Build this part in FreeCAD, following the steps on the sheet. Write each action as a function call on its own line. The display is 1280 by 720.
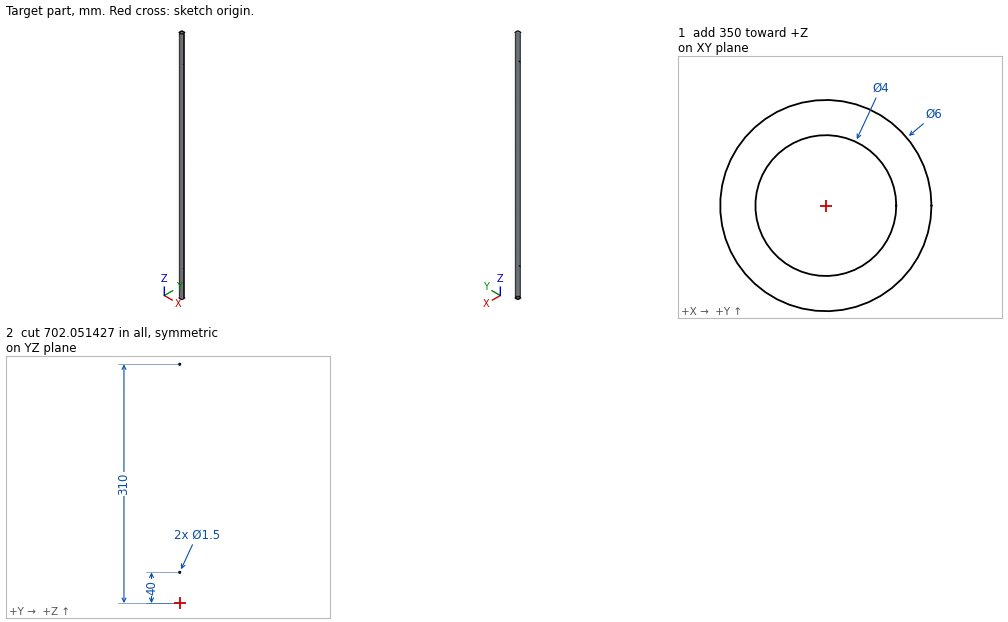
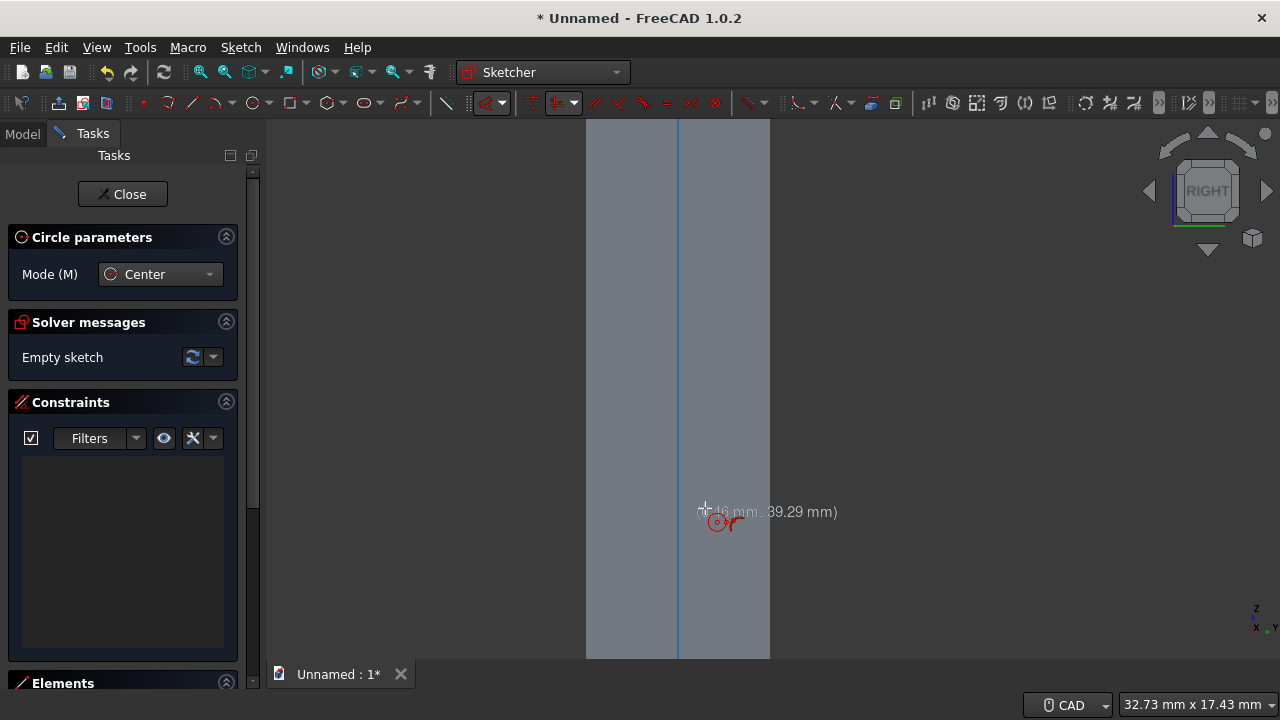
scroll(706, 536, down, 16)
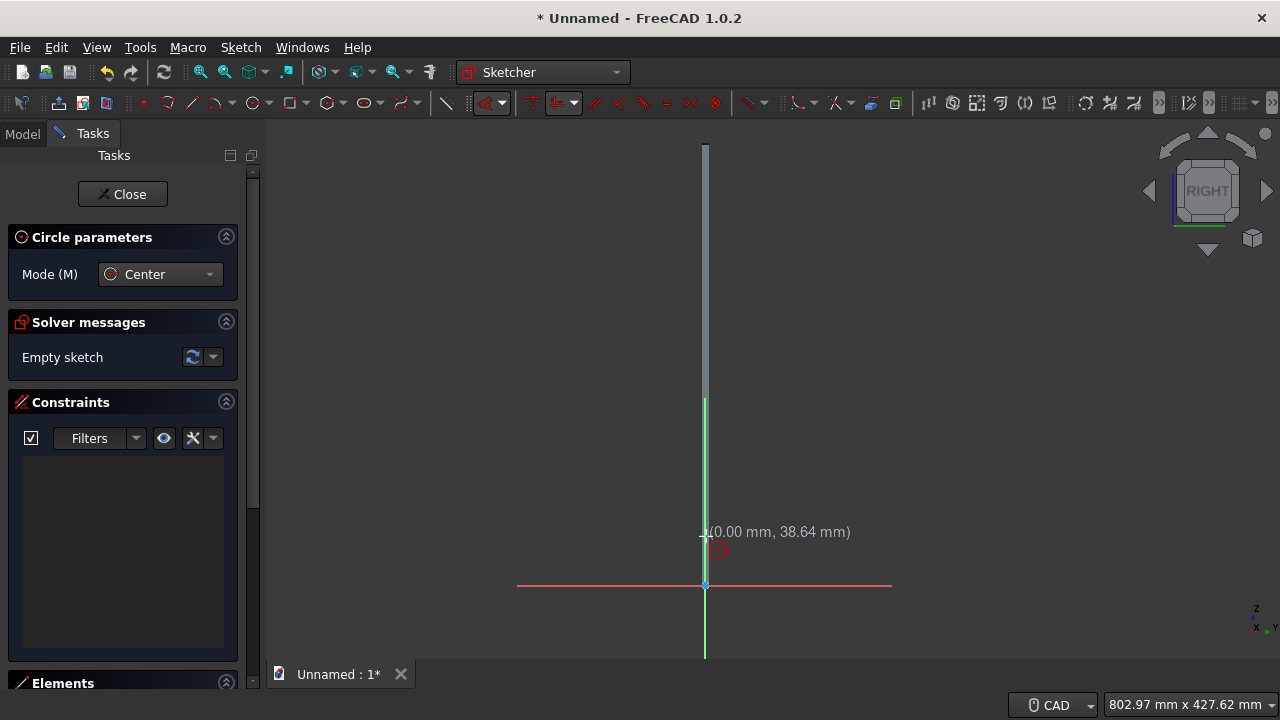
click(705, 535)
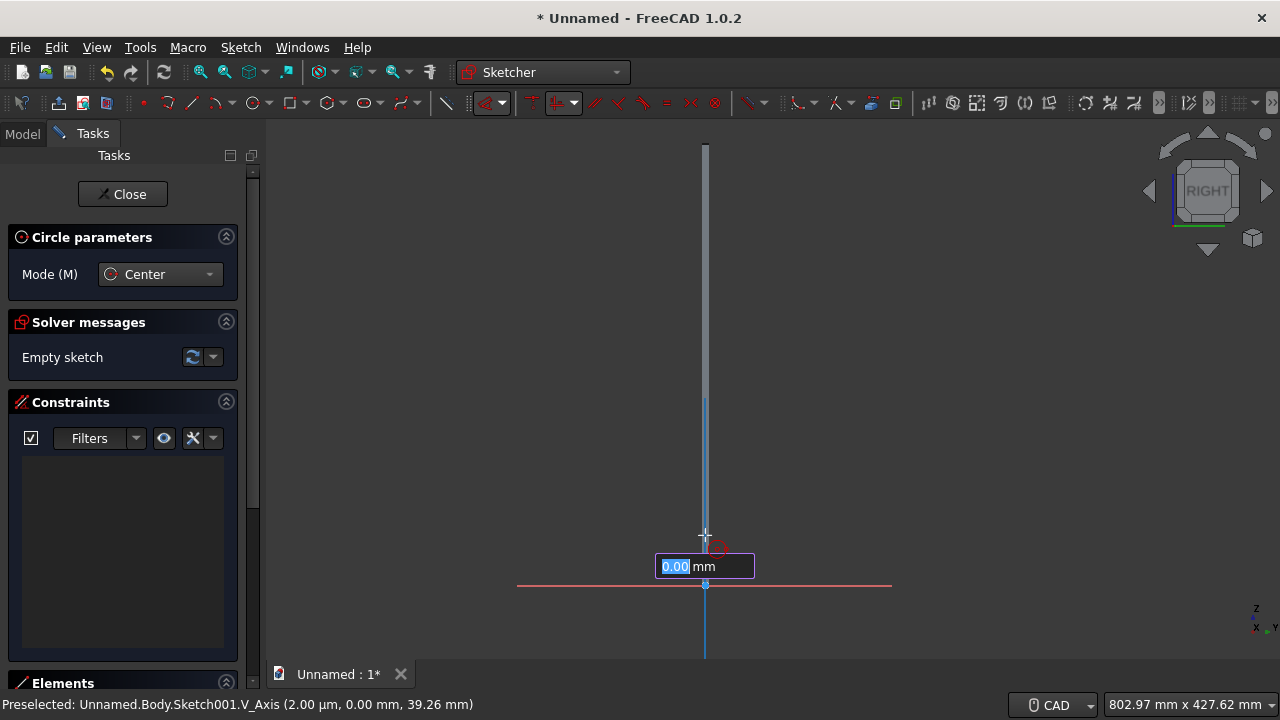
scroll(706, 535, up, 15)
move(701, 515)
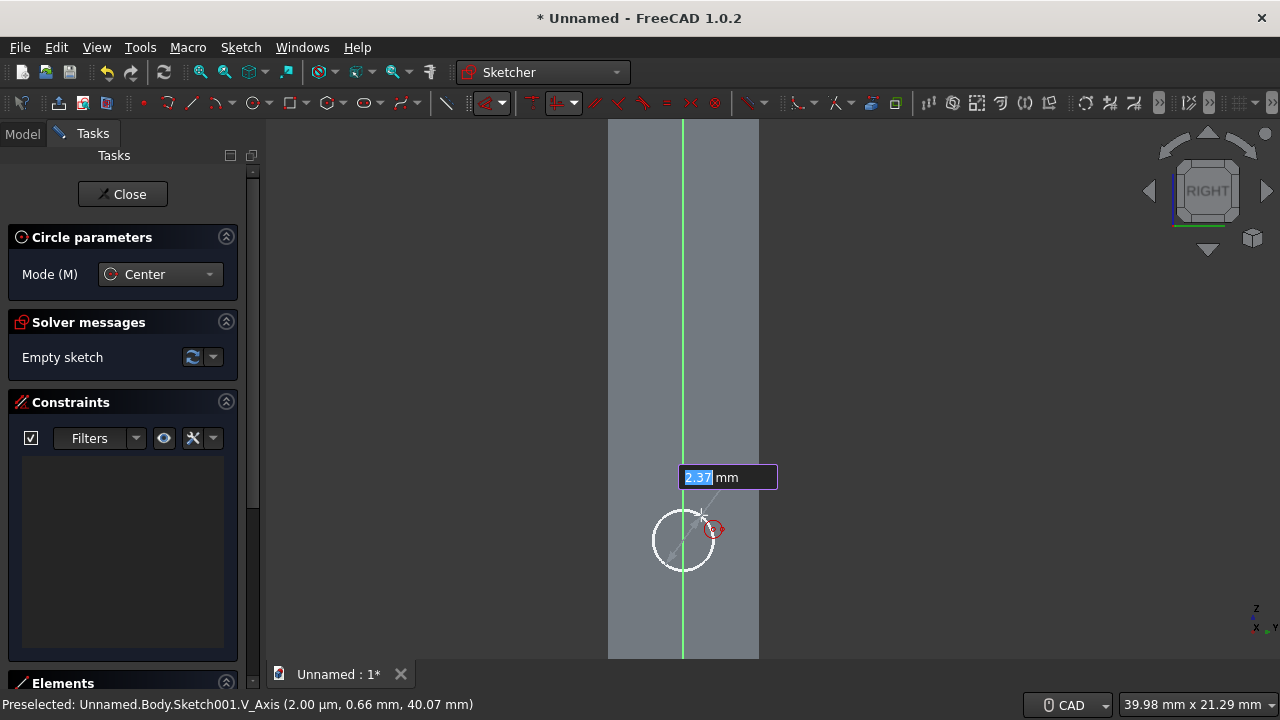
text(1.5)
key(Return)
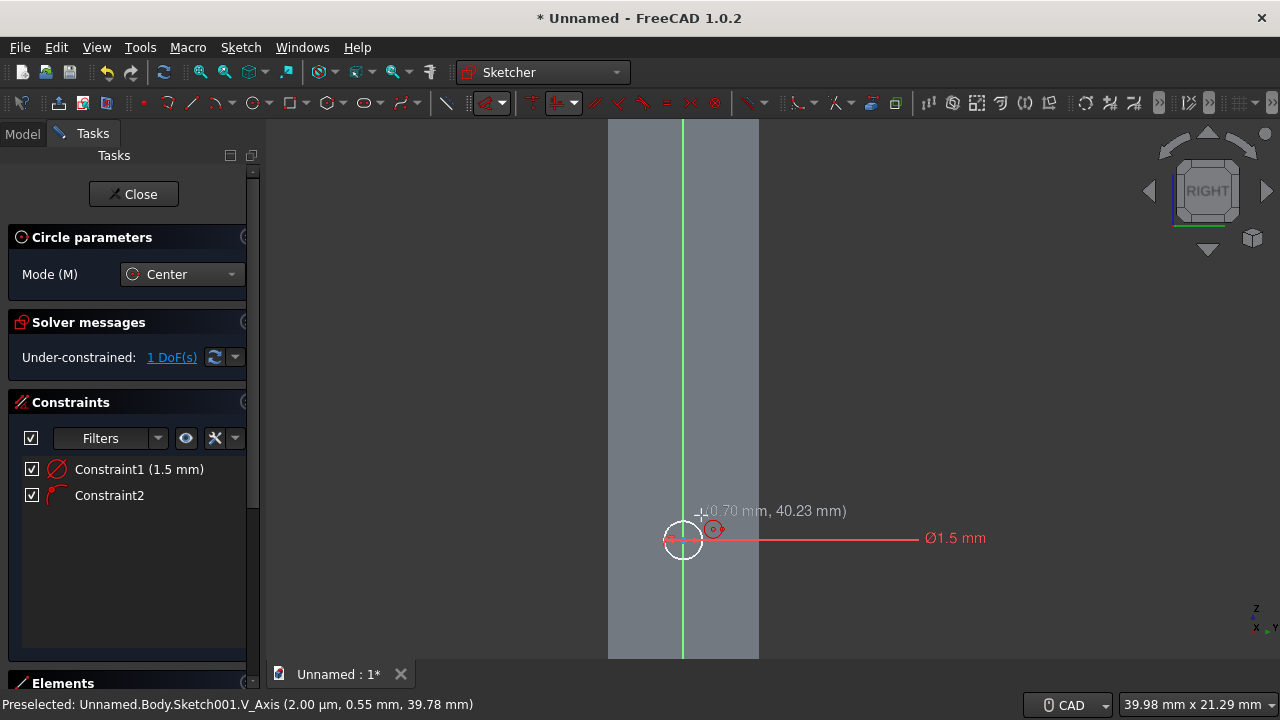
scroll(706, 535, down, 15)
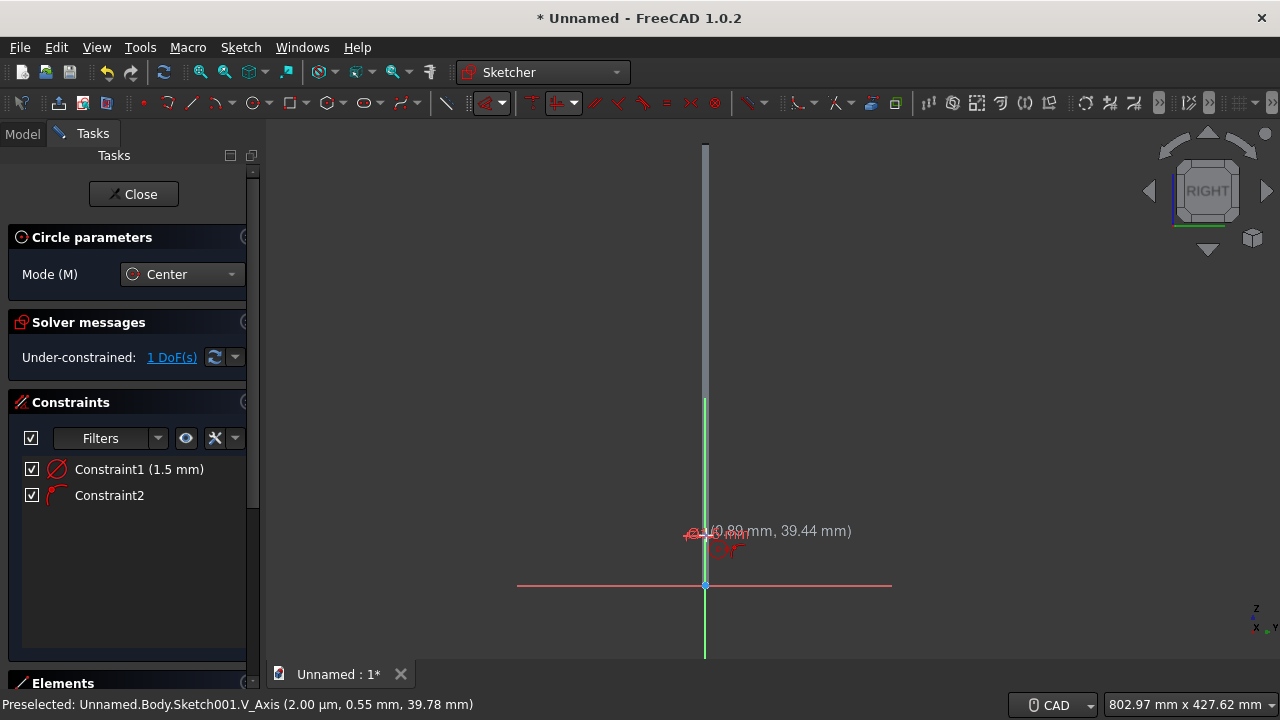
scroll(705, 194, up, 16)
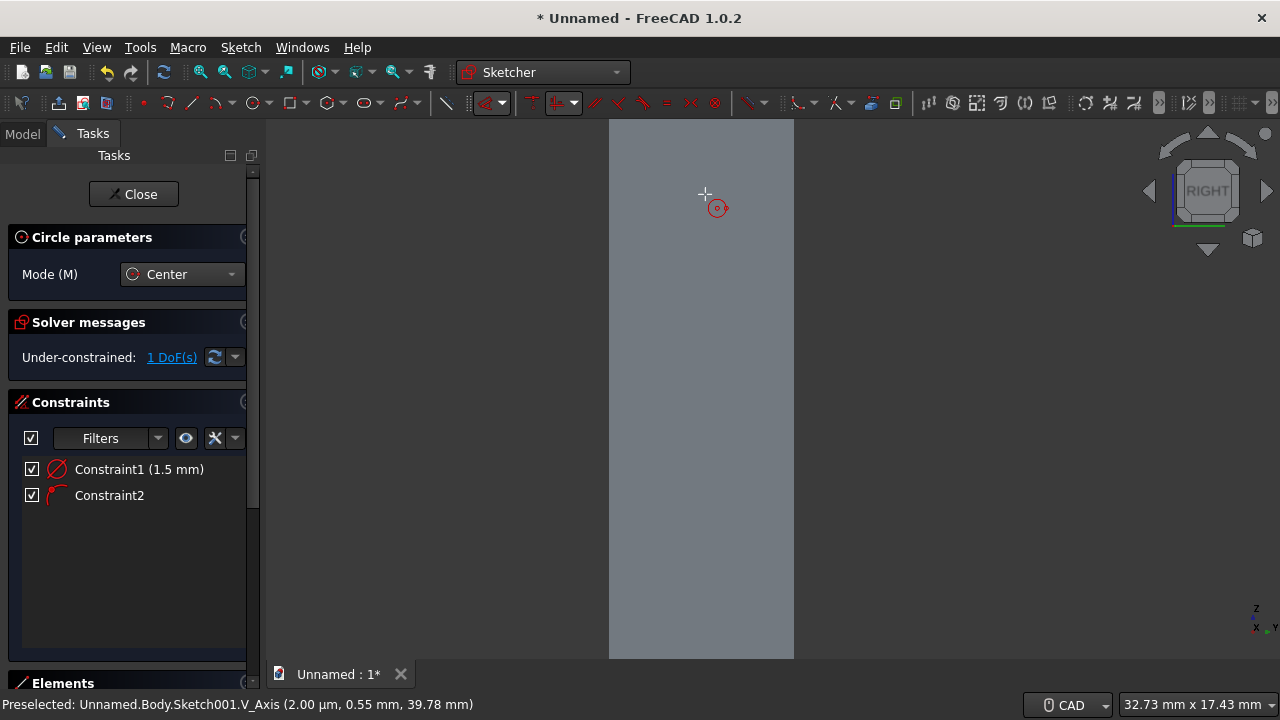
scroll(705, 194, down, 16)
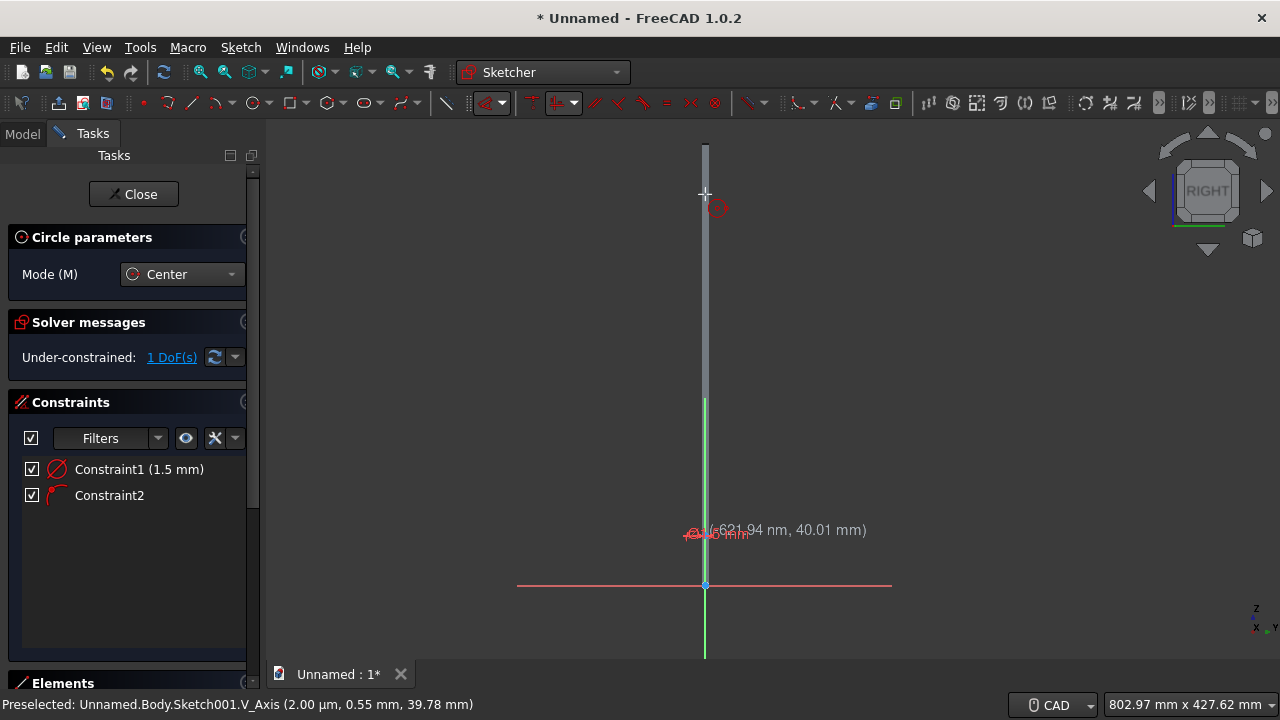
click(705, 194)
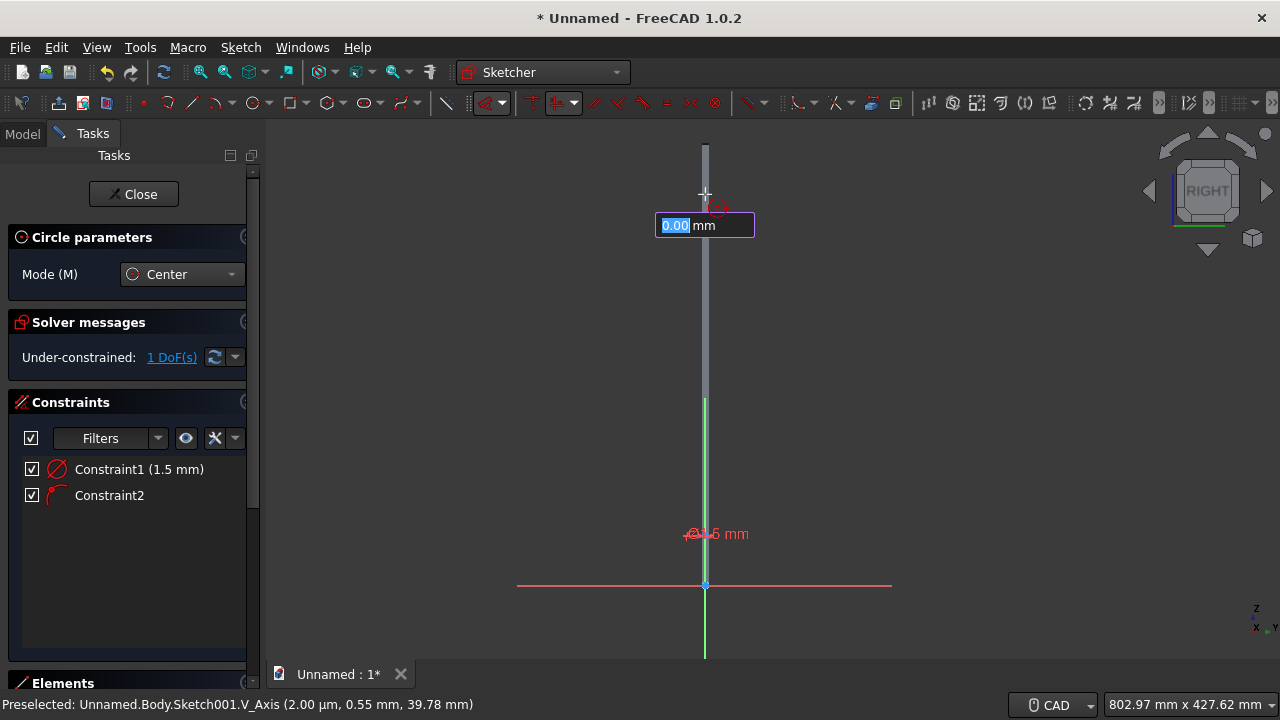
scroll(706, 194, up, 15)
move(701, 187)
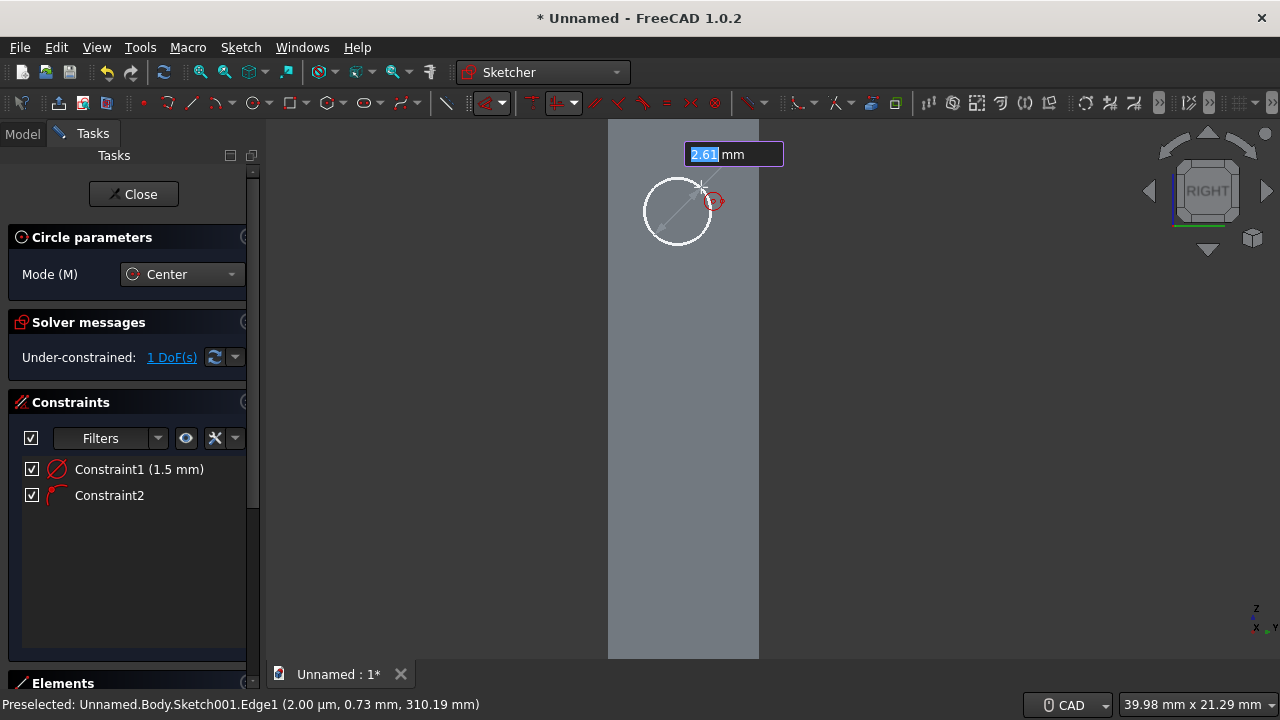
text(1.5)
key(Return)
key(Escape)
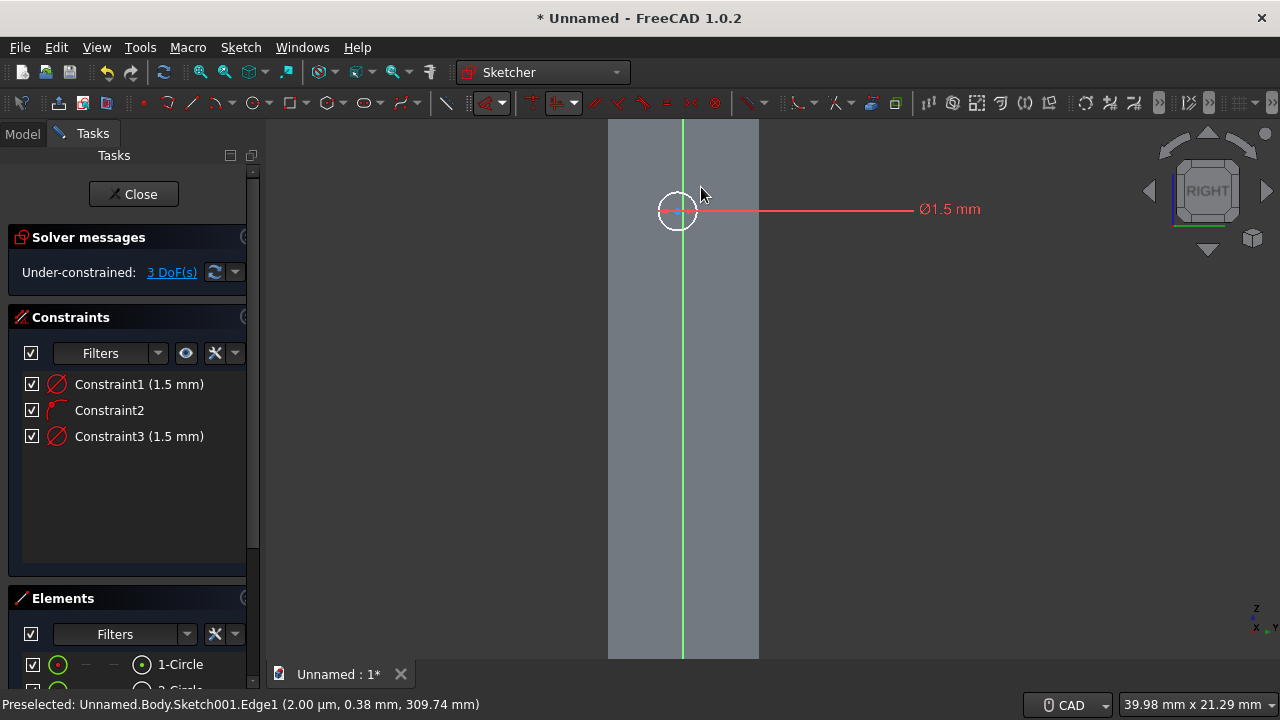
scroll(706, 194, down, 15)